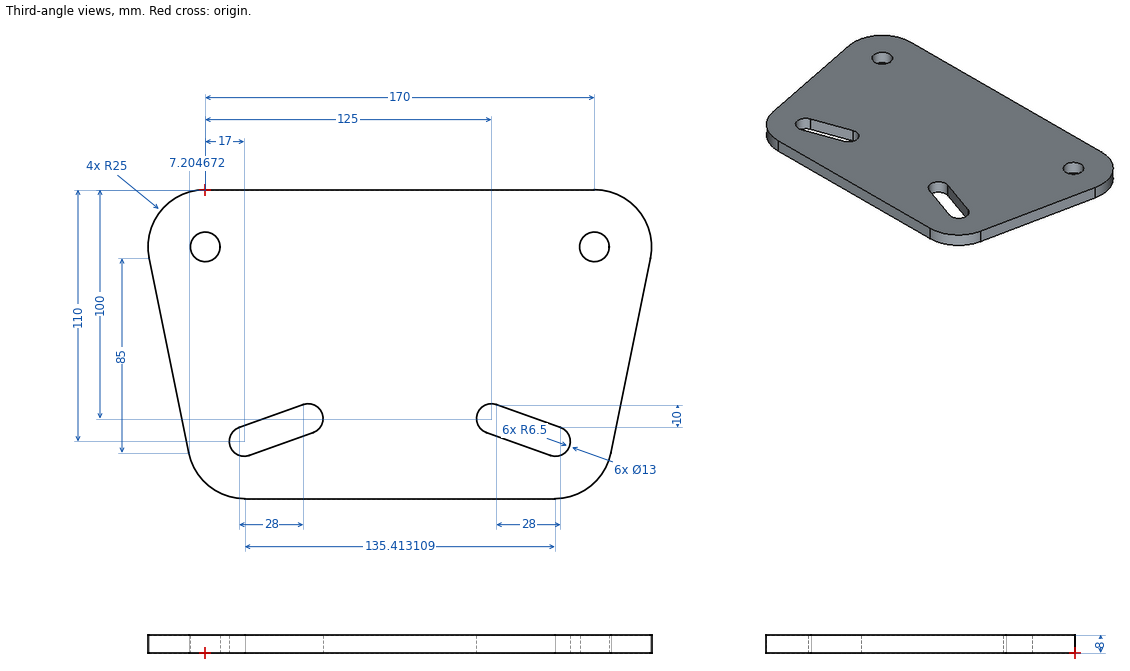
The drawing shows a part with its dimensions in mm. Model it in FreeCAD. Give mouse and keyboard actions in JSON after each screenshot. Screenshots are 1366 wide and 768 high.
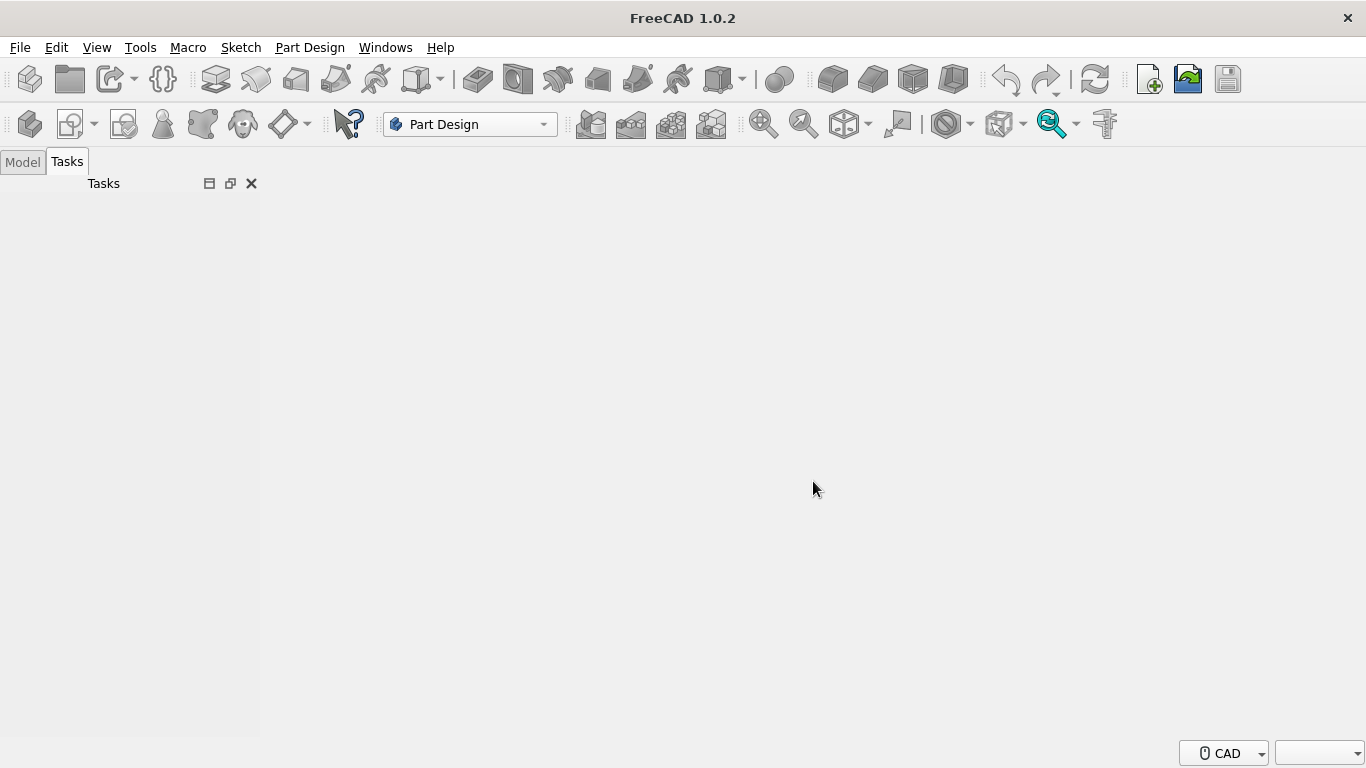
{"action": "left_click", "coordinate": [1148, 80]}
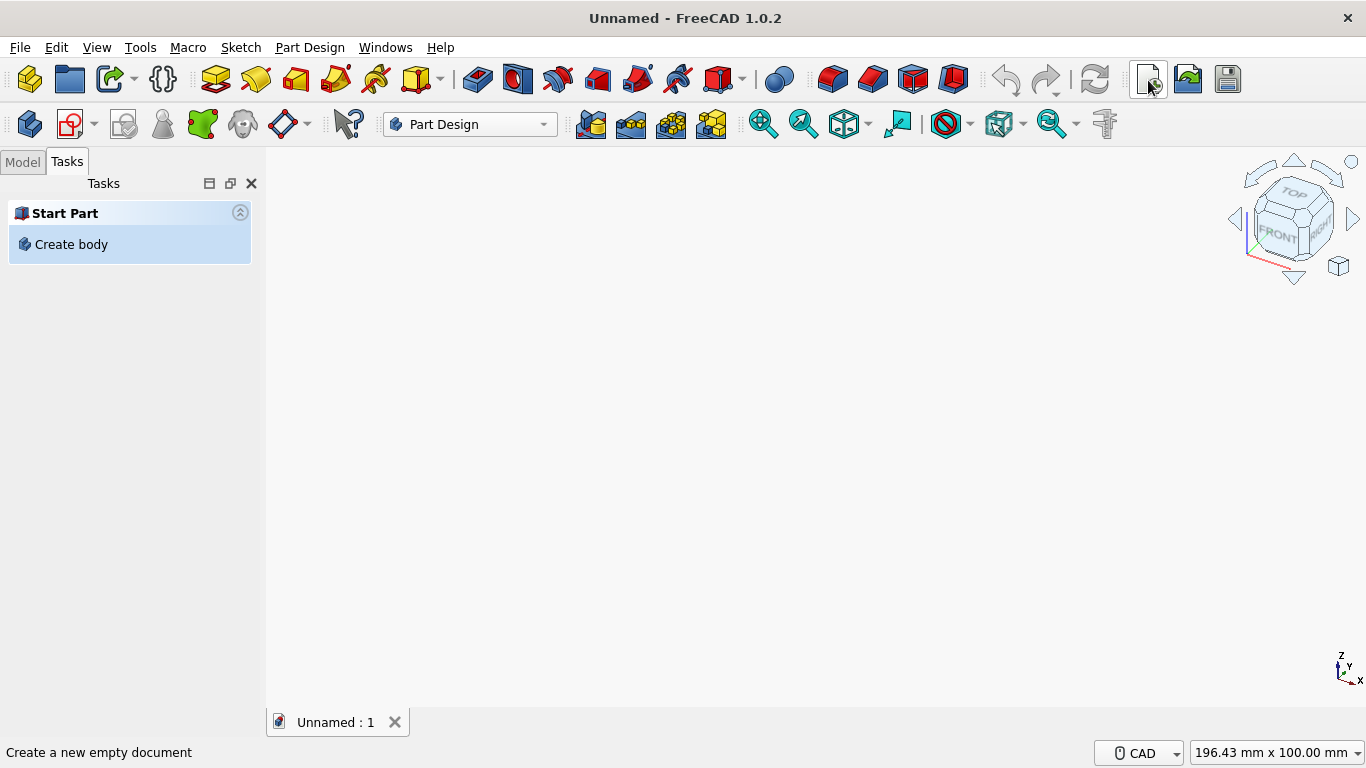
{"action": "left_click", "coordinate": [70, 124]}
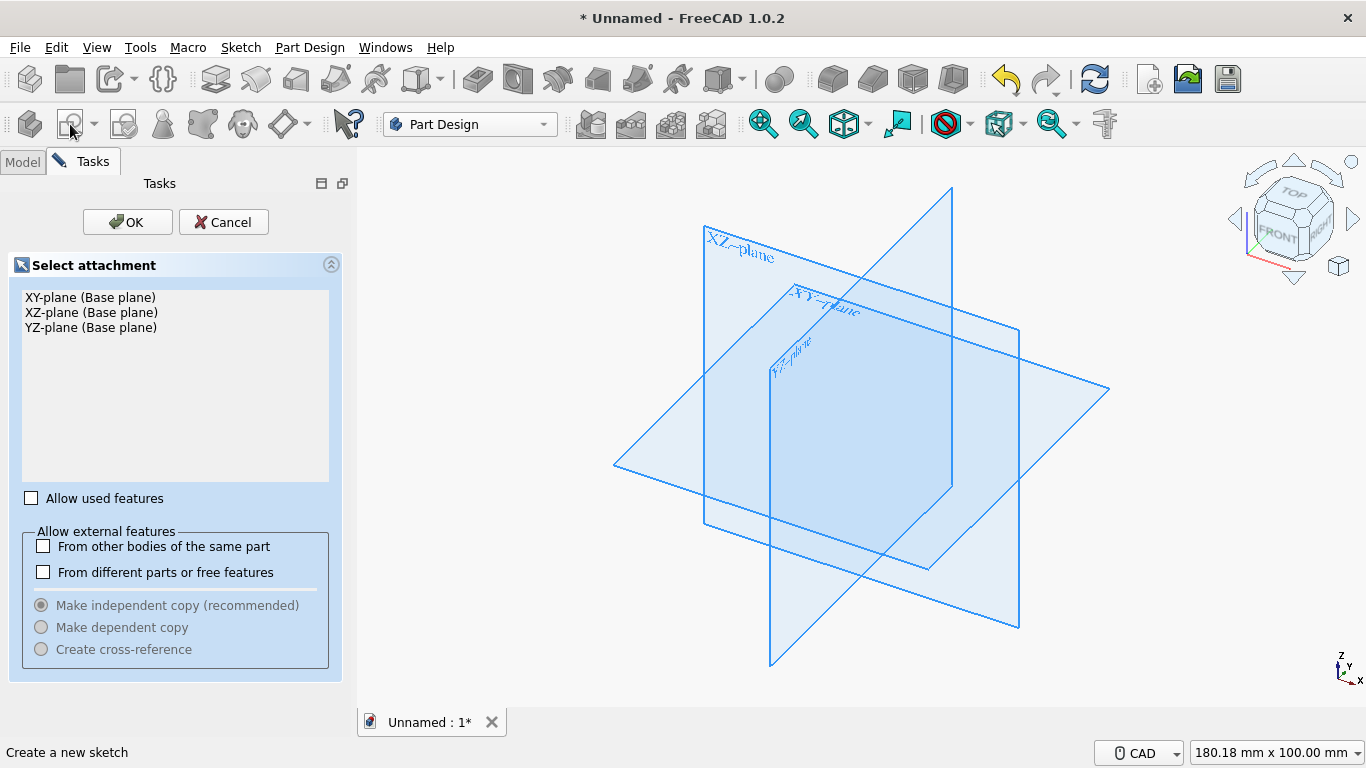
{"action": "left_click", "coordinate": [82, 298]}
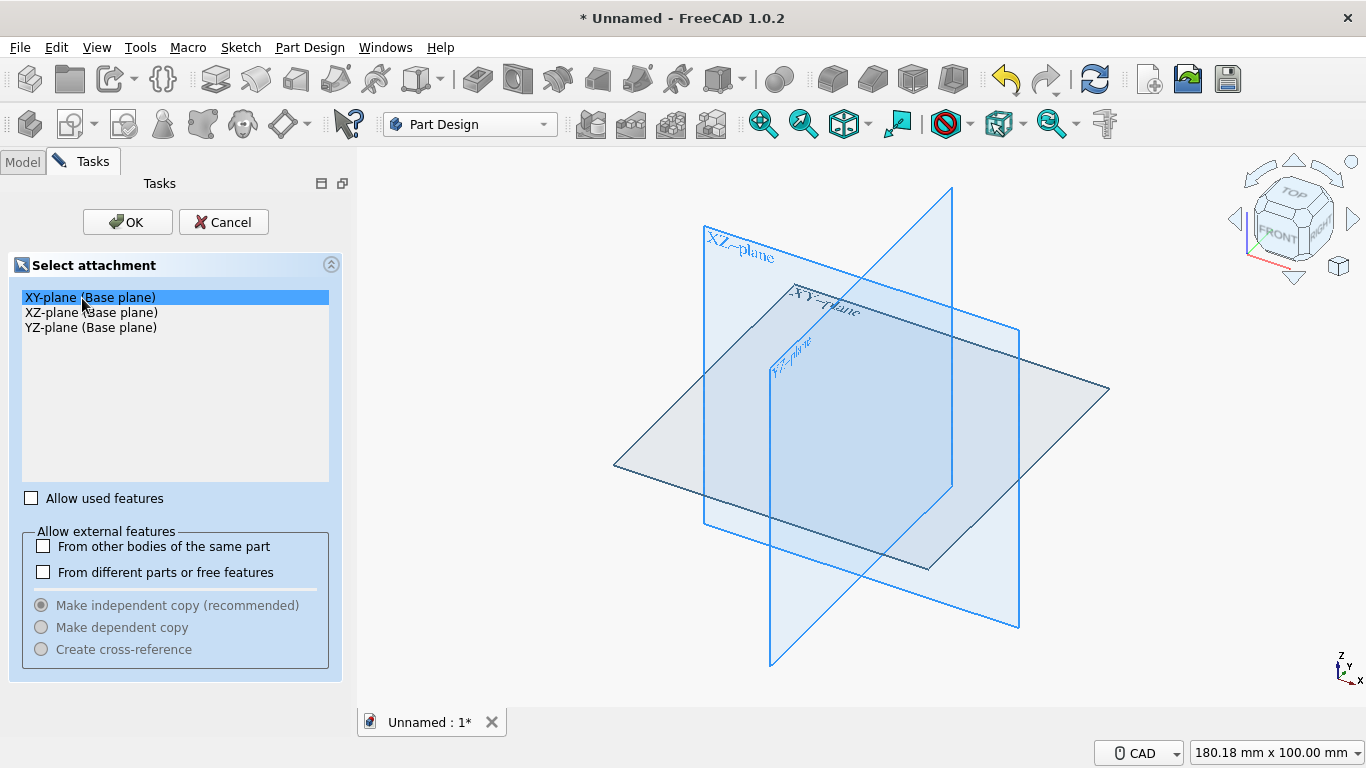
{"action": "left_click", "coordinate": [128, 222]}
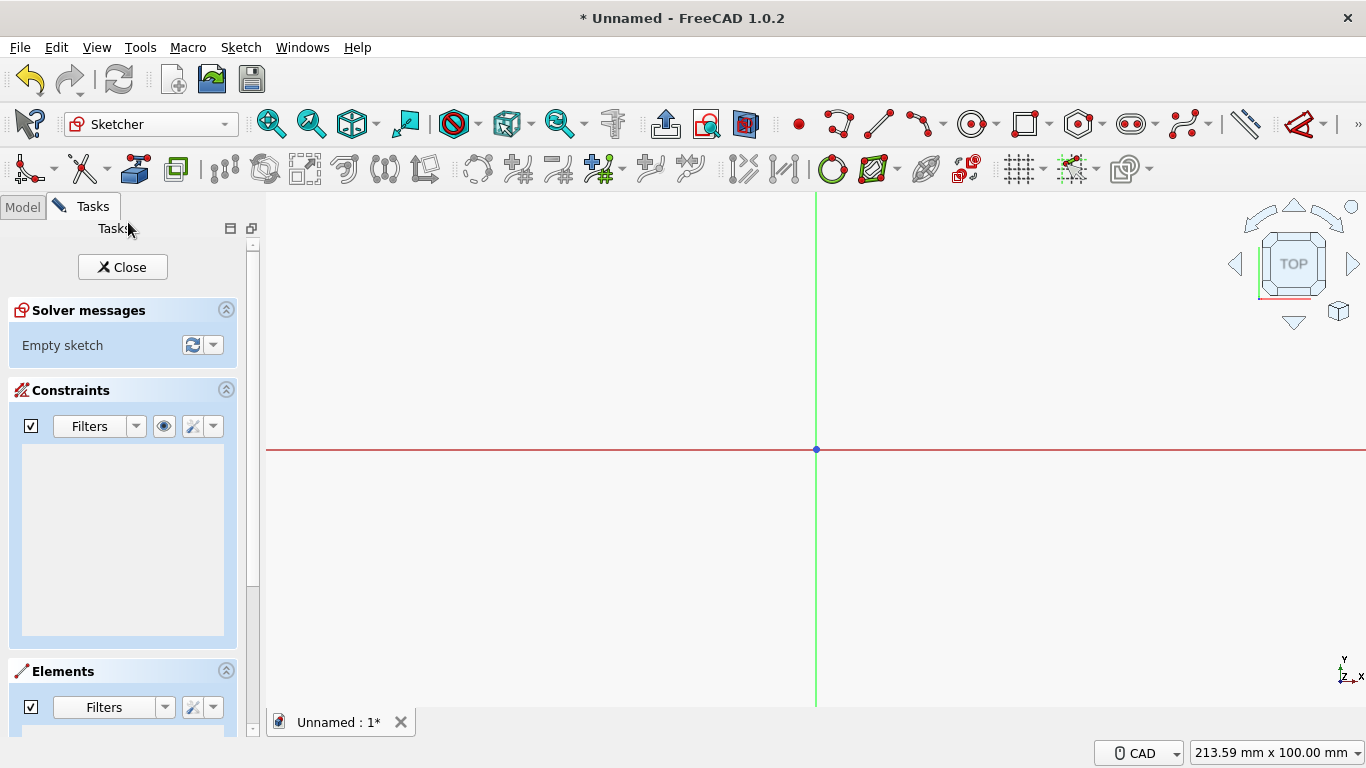
{"action": "scroll", "coordinate": [334, 220], "scroll_direction": "down", "scroll_amount": 4}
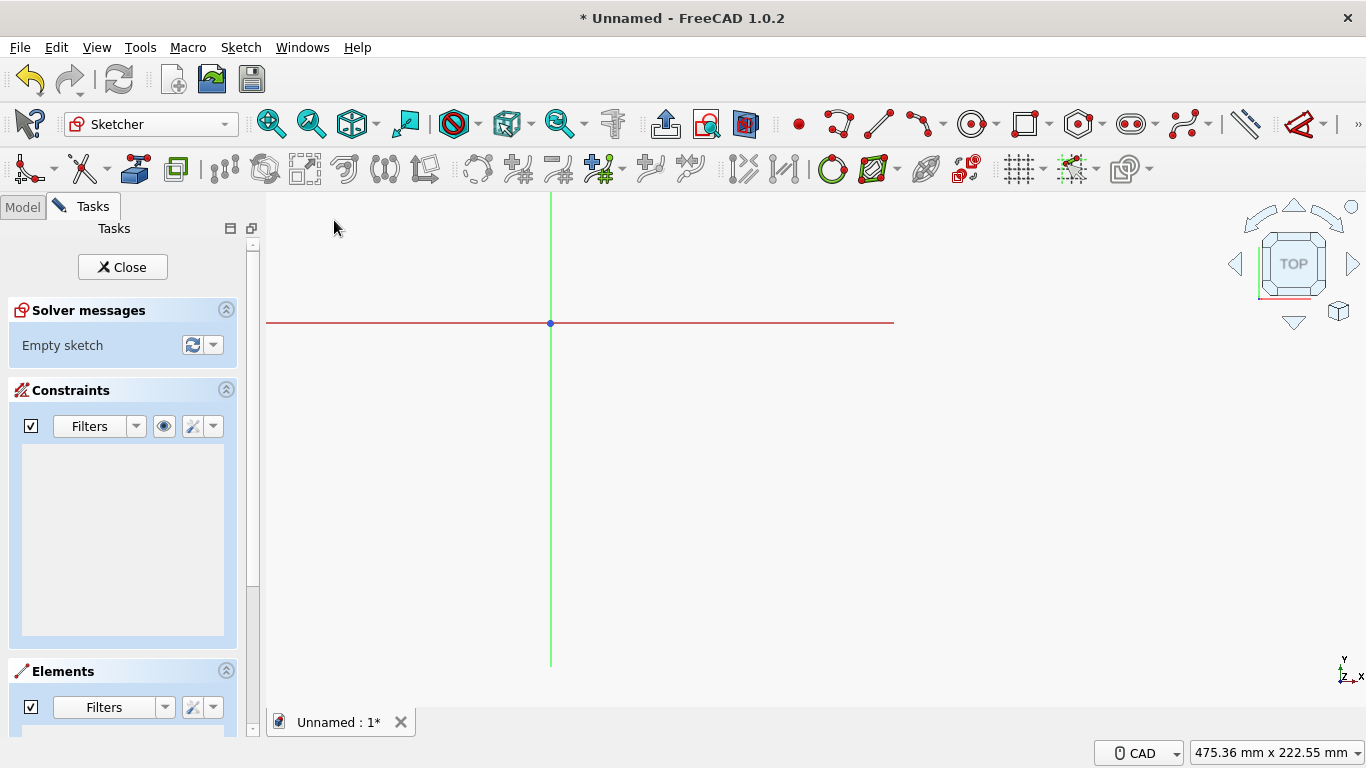
{"action": "left_click", "coordinate": [880, 124]}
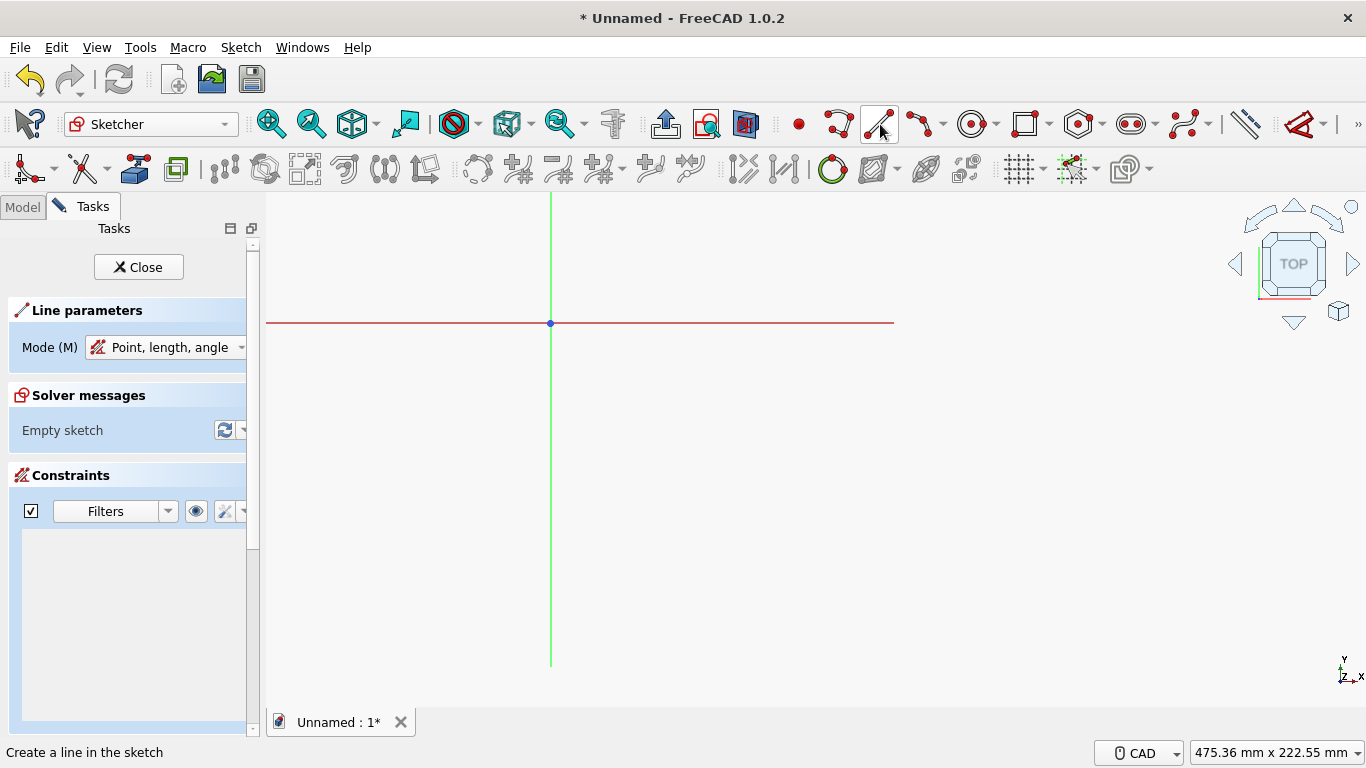
{"action": "left_click", "coordinate": [944, 323]}
{"action": "left_click", "coordinate": [551, 323]}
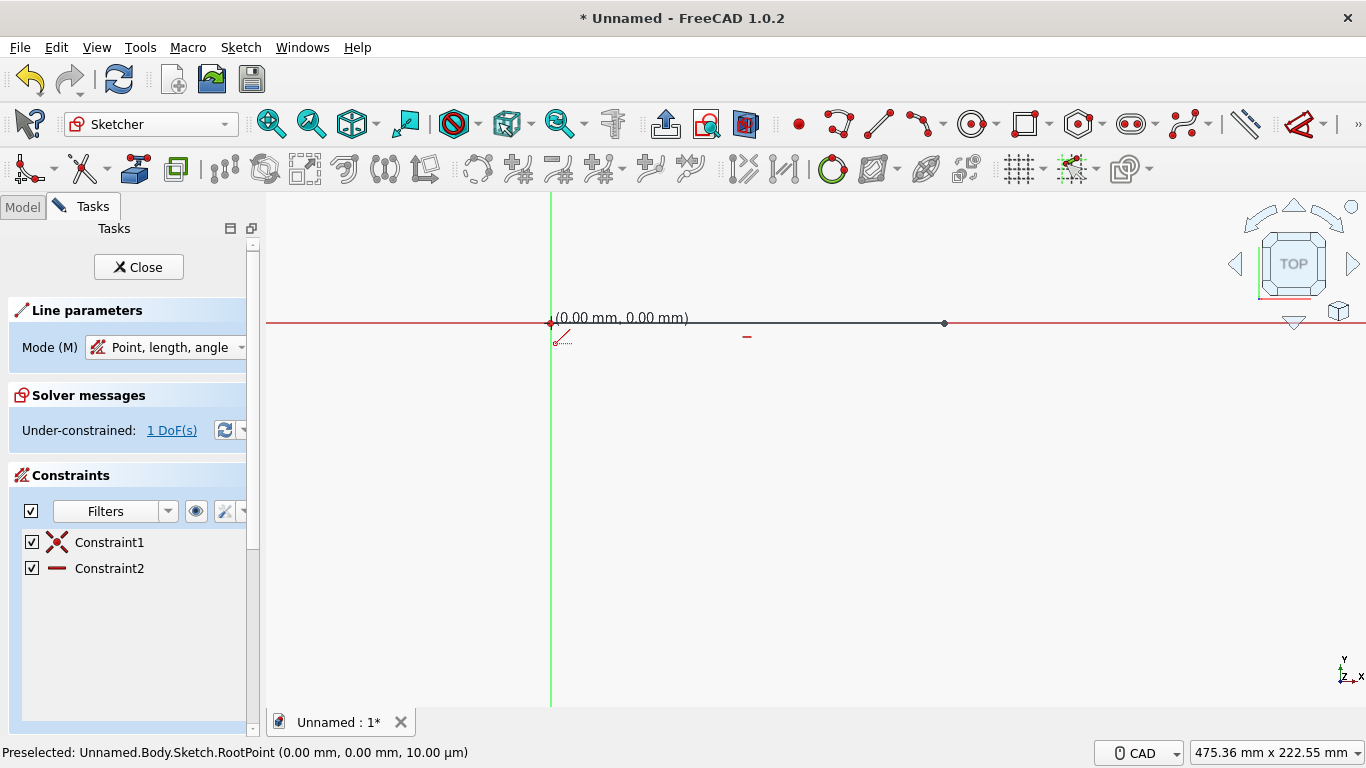
{"action": "left_click", "coordinate": [494, 393]}
{"action": "left_click", "coordinate": [534, 589]}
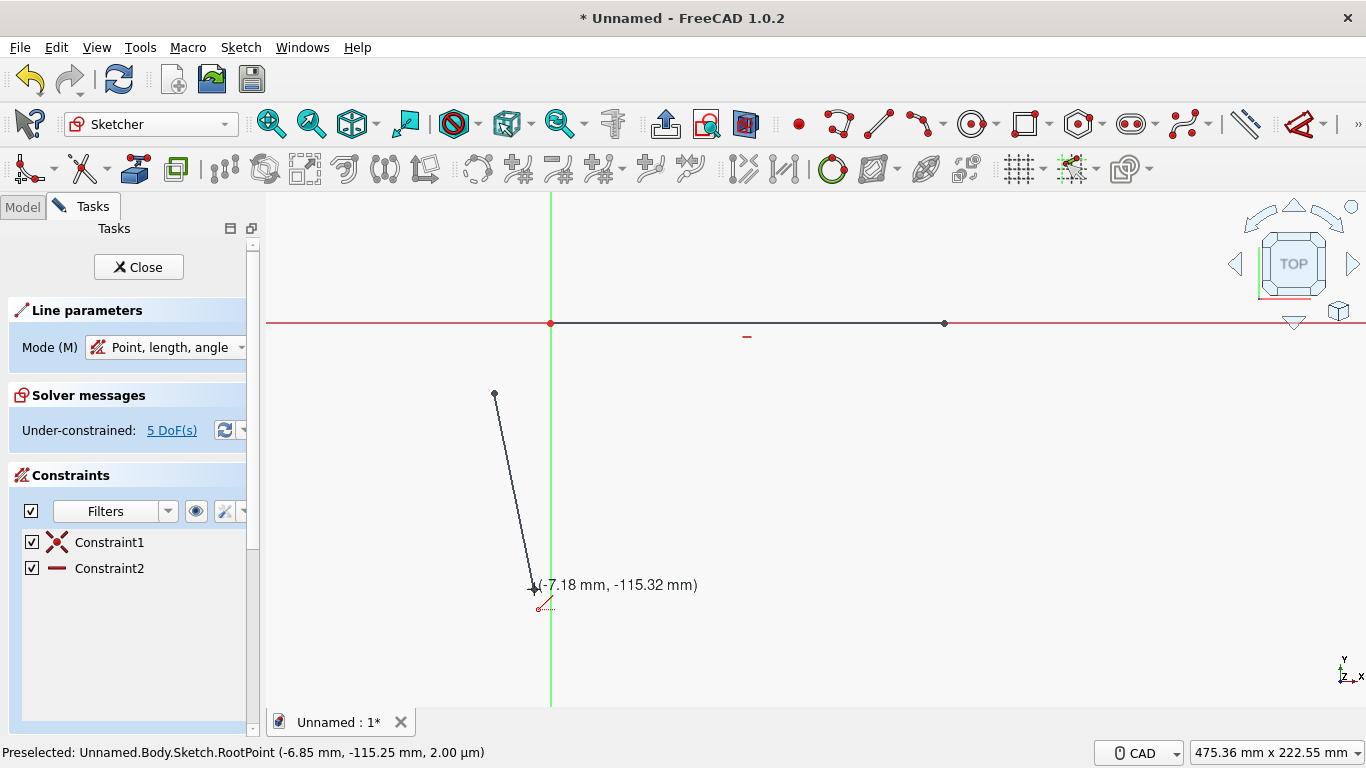
{"action": "left_click", "coordinate": [591, 636]}
{"action": "left_click", "coordinate": [904, 636]}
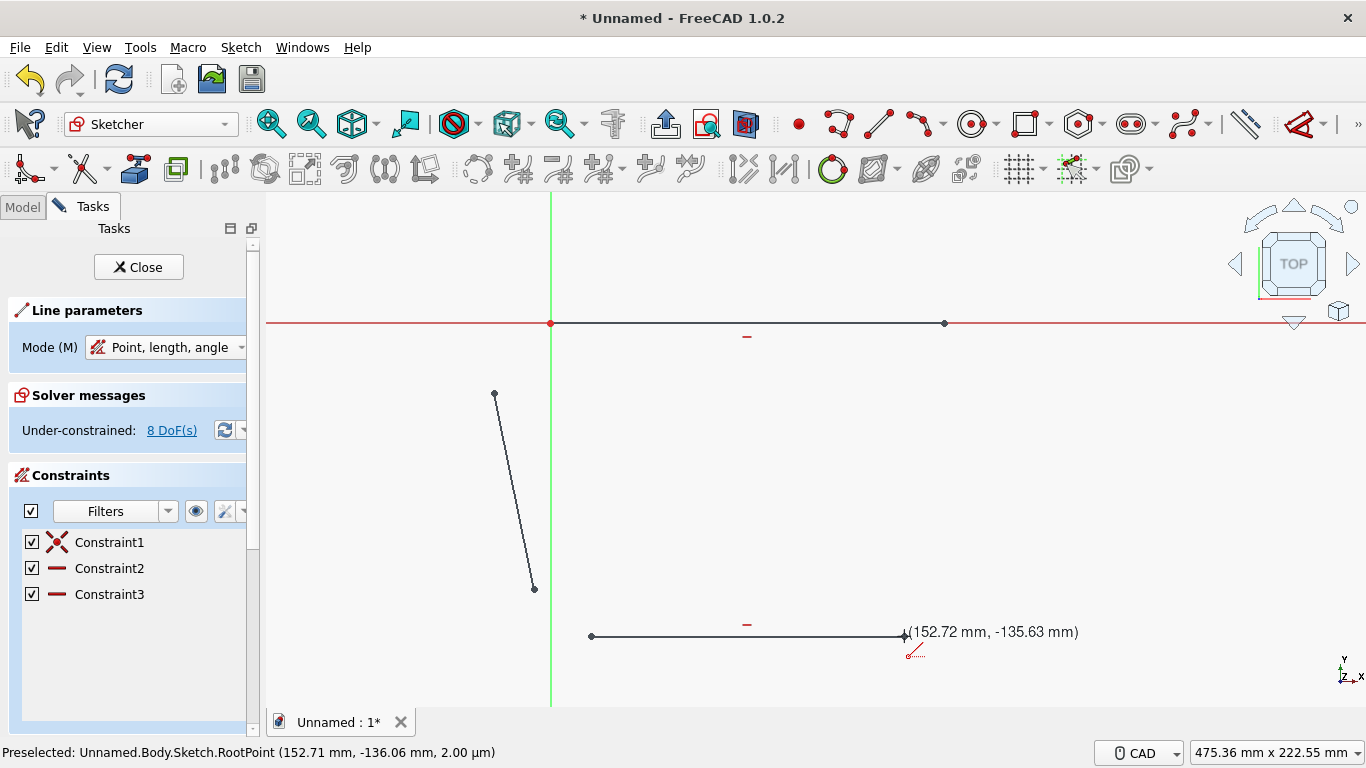
{"action": "left_click", "coordinate": [961, 589]}
{"action": "left_click", "coordinate": [1001, 393]}